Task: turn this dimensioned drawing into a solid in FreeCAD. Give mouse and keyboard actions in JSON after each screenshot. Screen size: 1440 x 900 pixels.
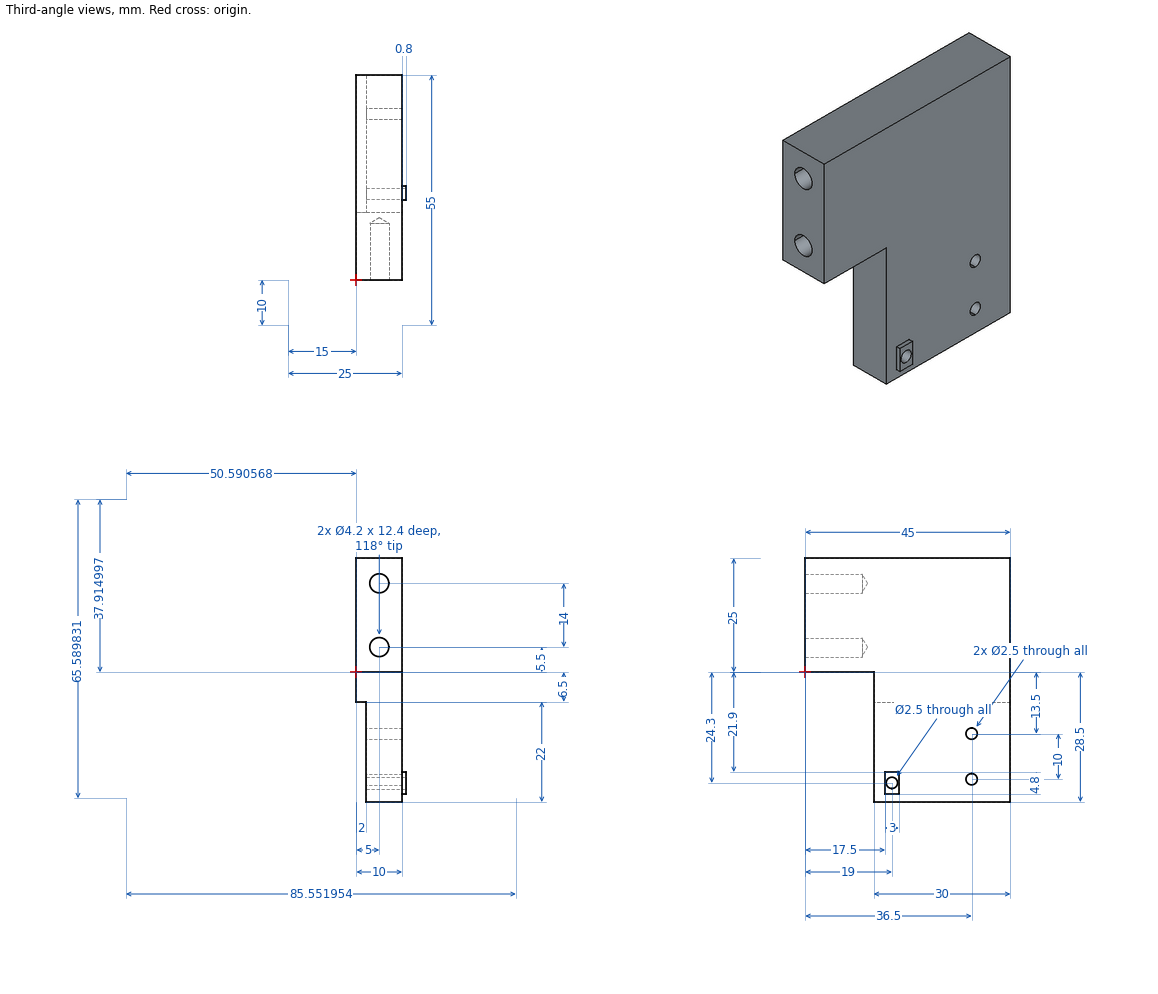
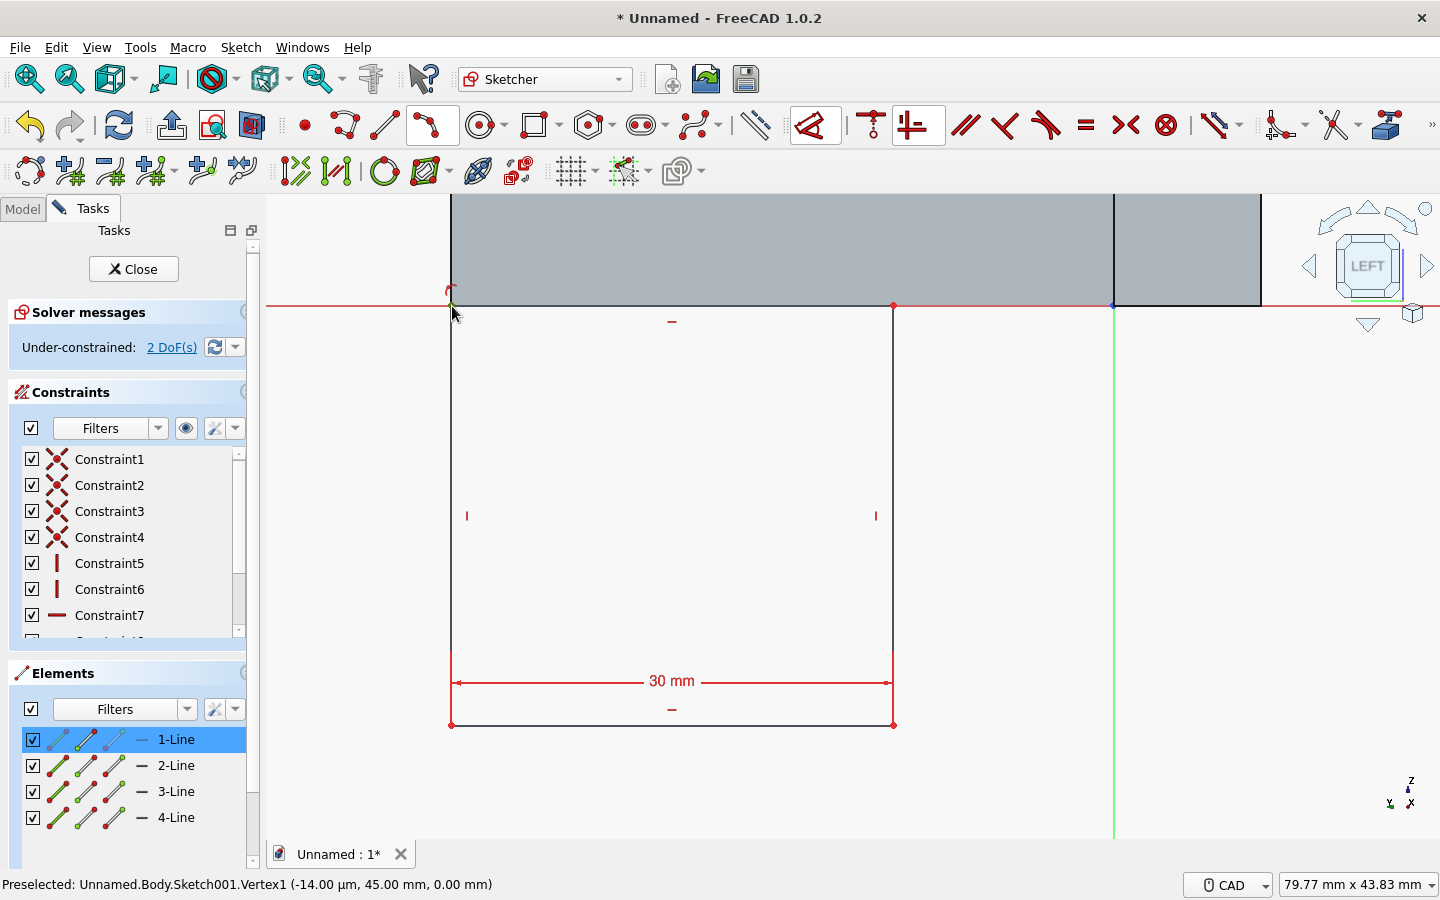
{"action": "key", "text": "l"}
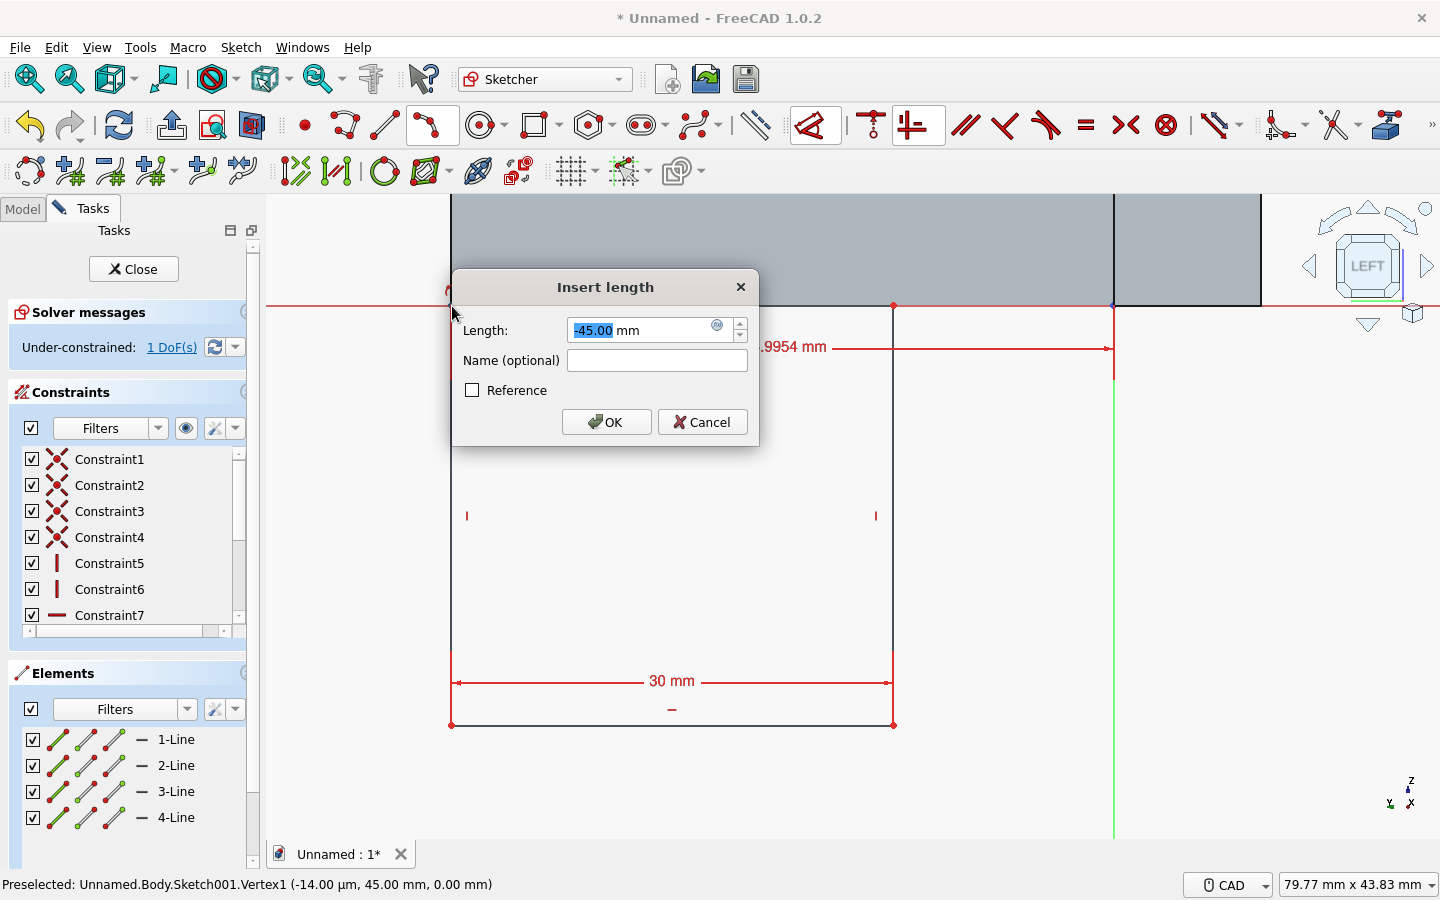
{"action": "type", "text": "-45"}
{"action": "key", "text": "Return"}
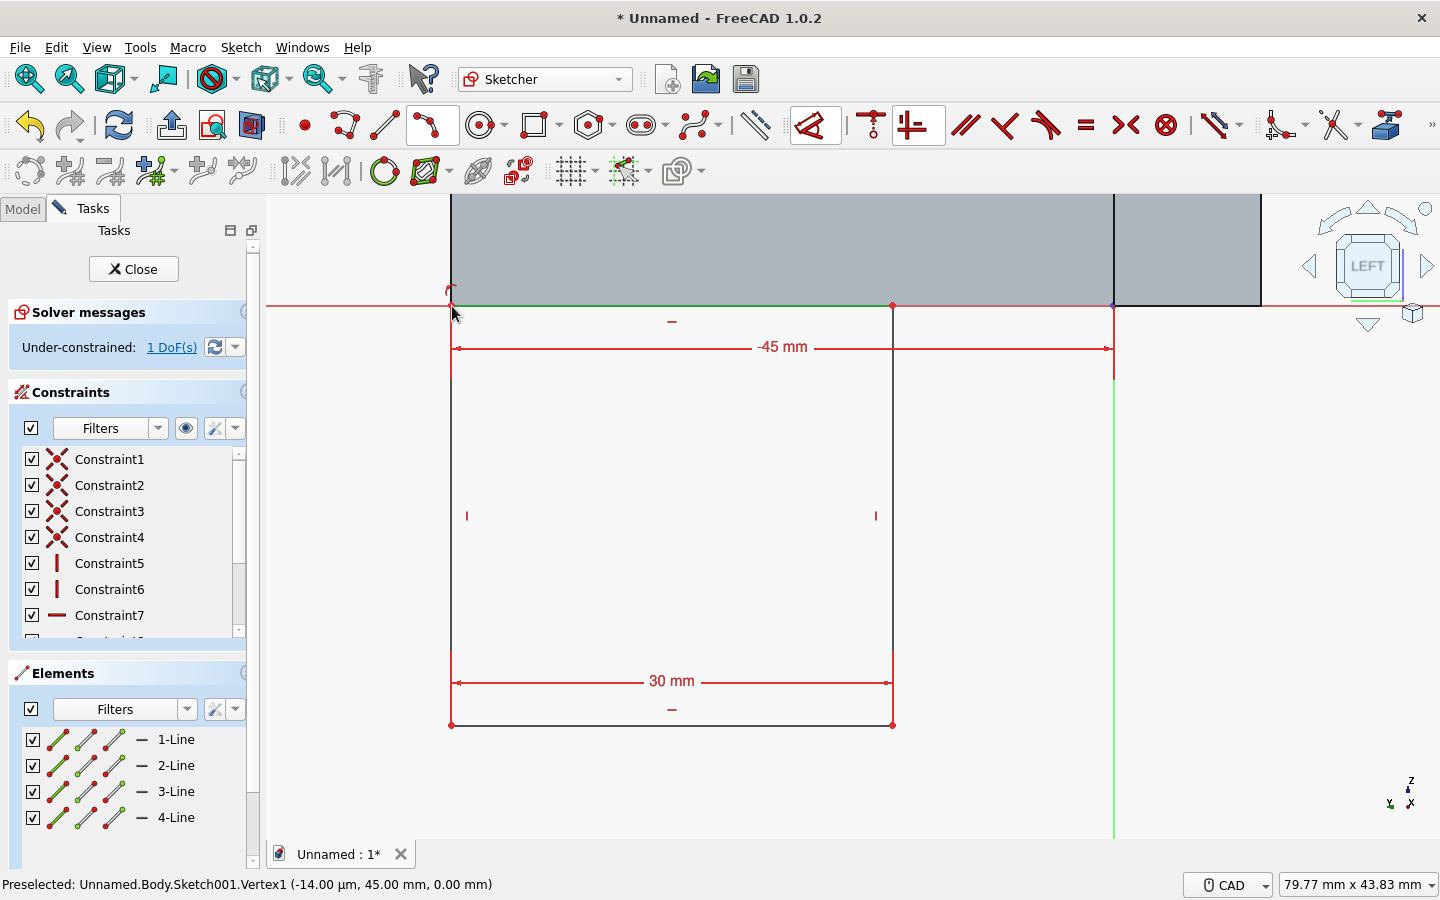
{"action": "left_click", "coordinate": [451, 432]}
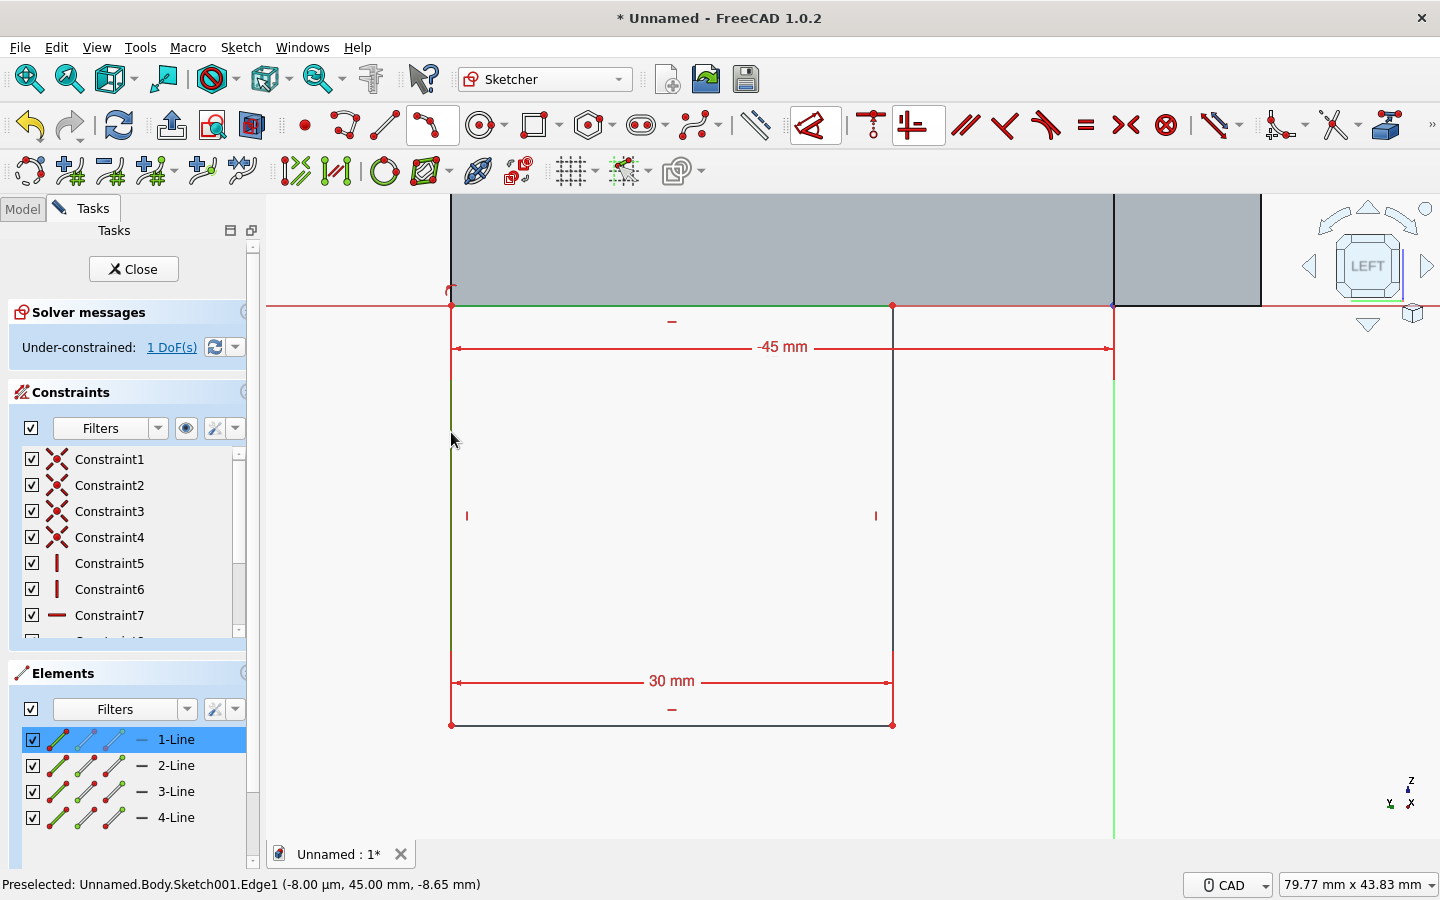
{"action": "key", "text": "i"}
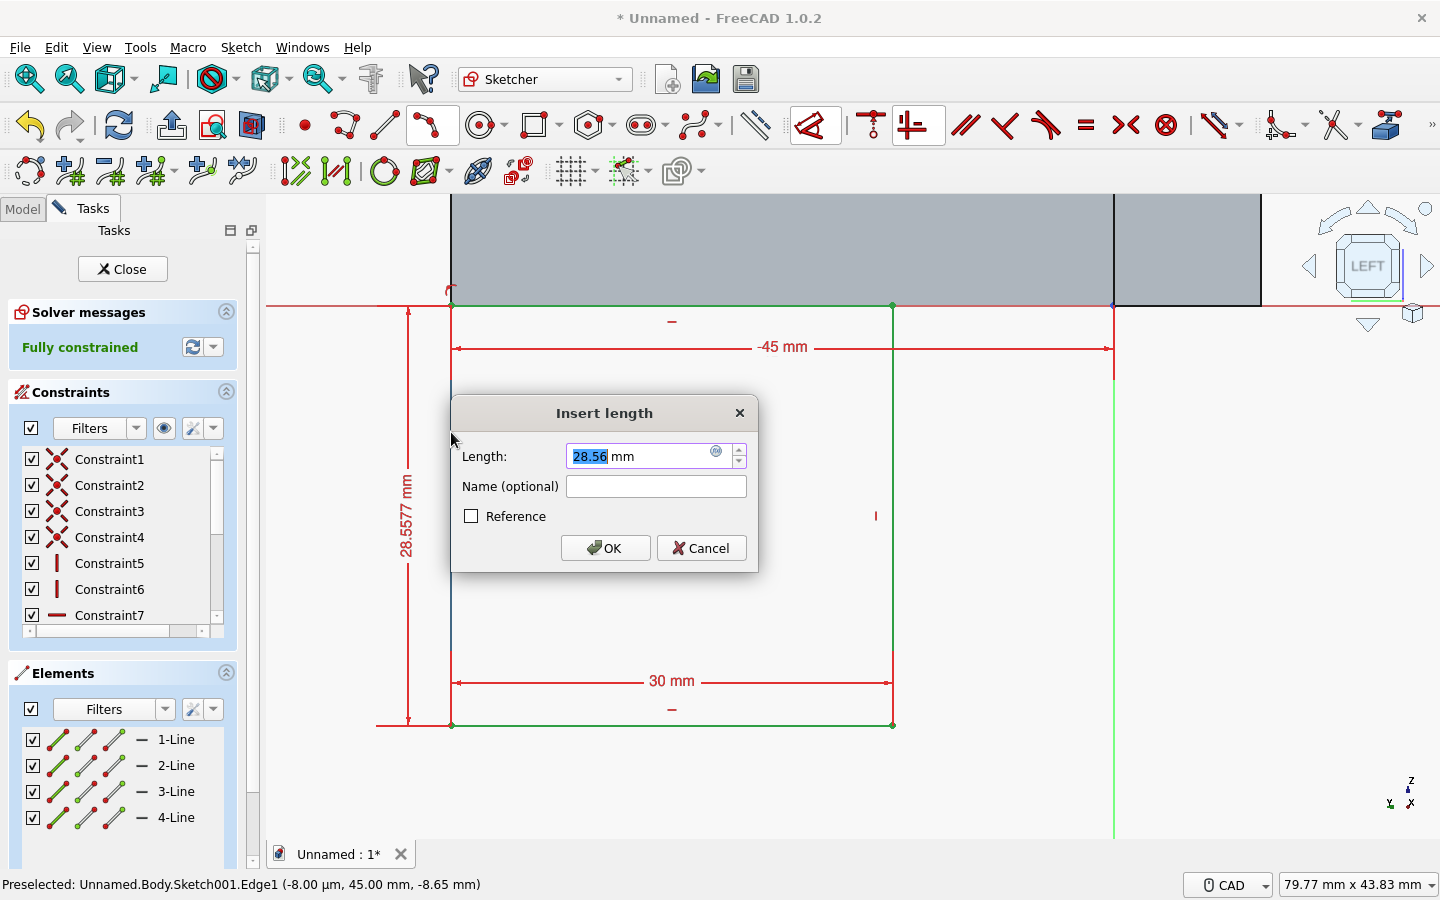
{"action": "type", "text": "28.5"}
{"action": "key", "text": "Return"}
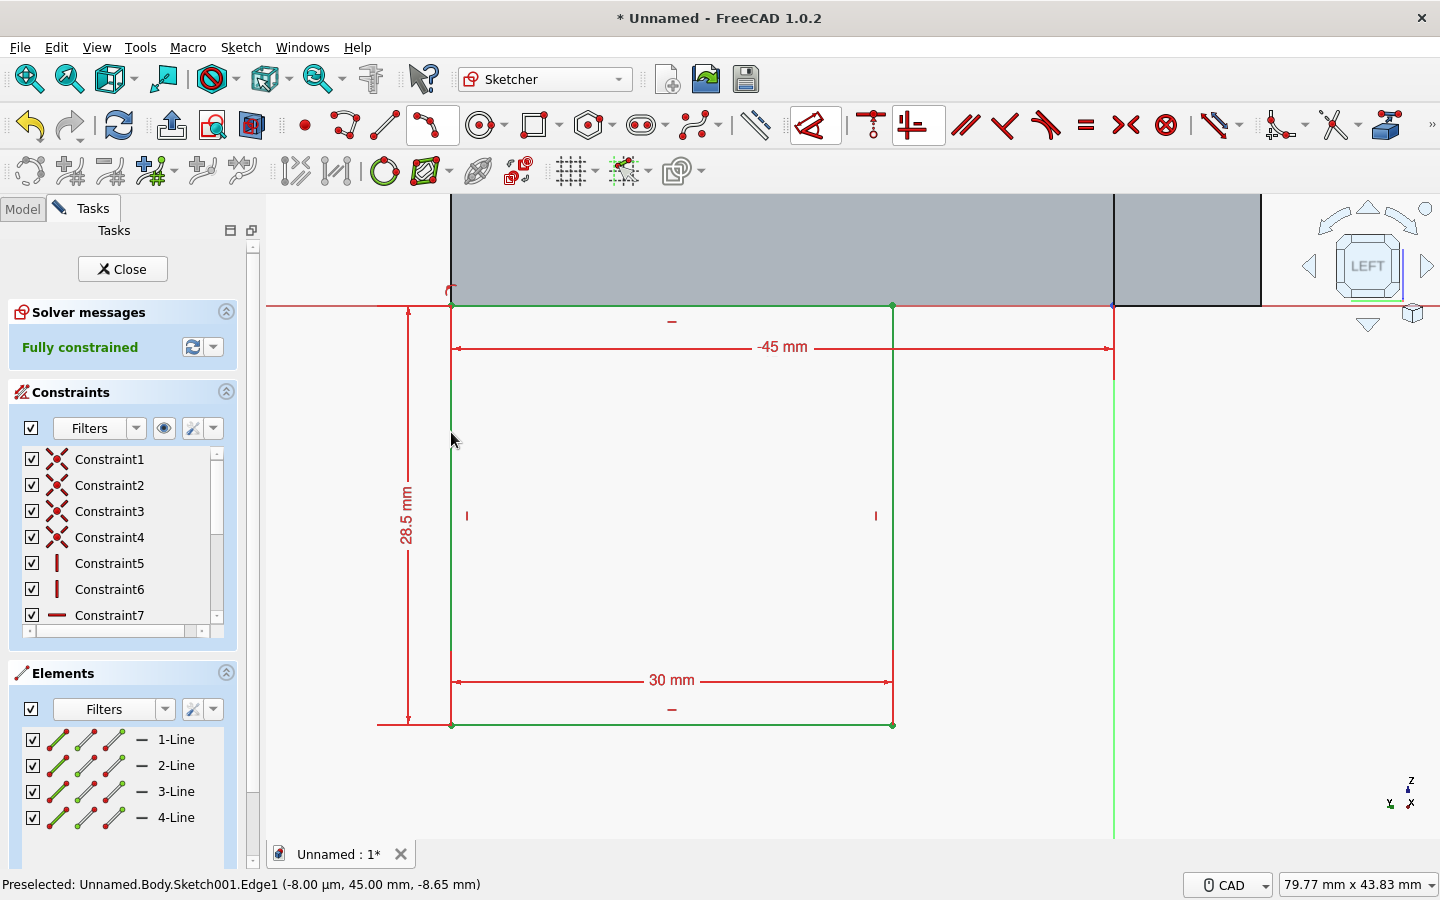
{"action": "left_click", "coordinate": [123, 269]}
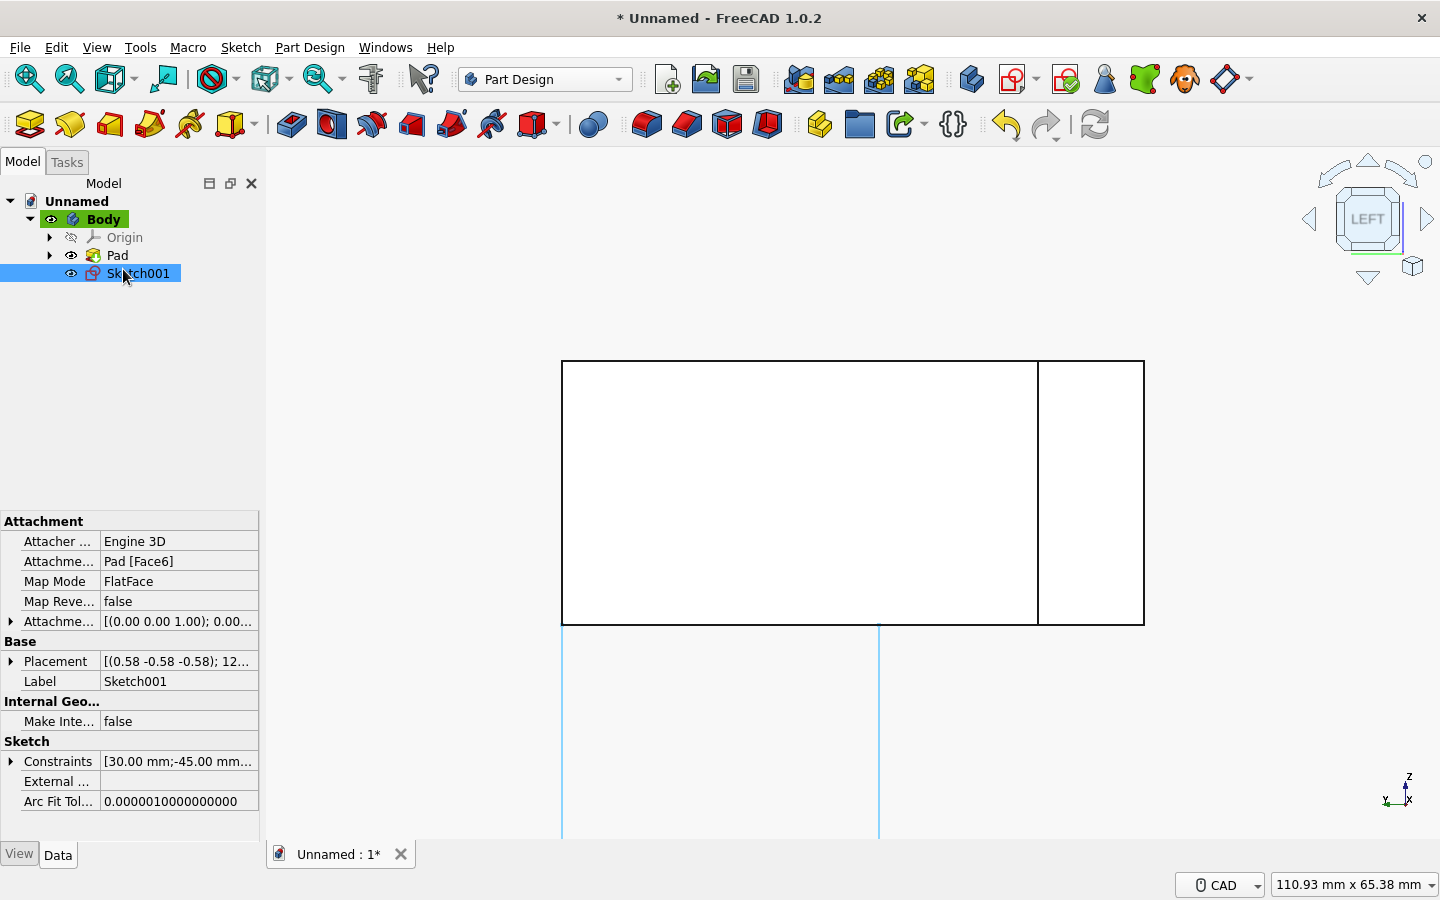
{"action": "left_click", "coordinate": [30, 124]}